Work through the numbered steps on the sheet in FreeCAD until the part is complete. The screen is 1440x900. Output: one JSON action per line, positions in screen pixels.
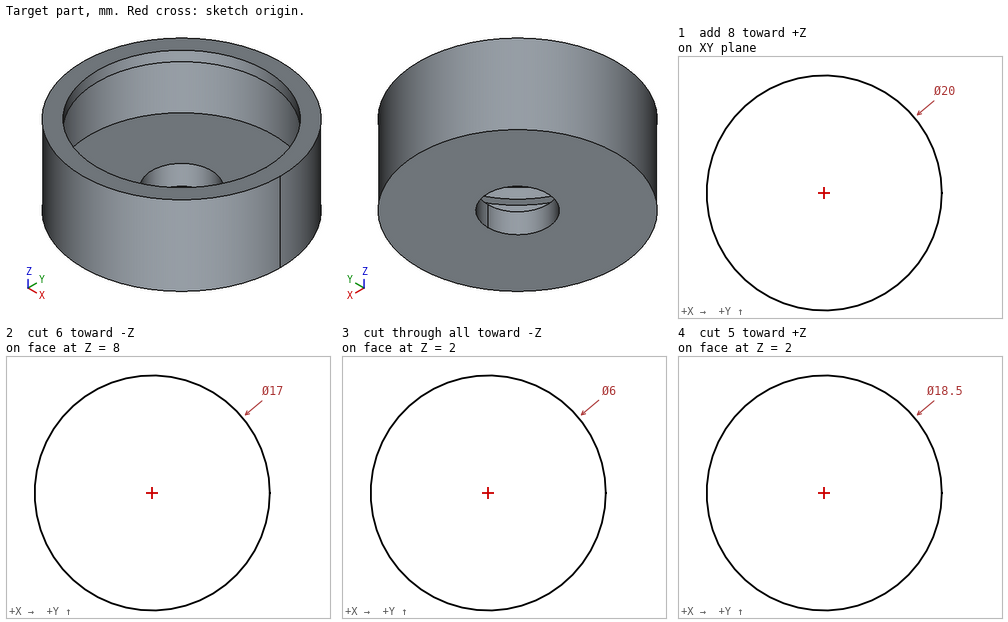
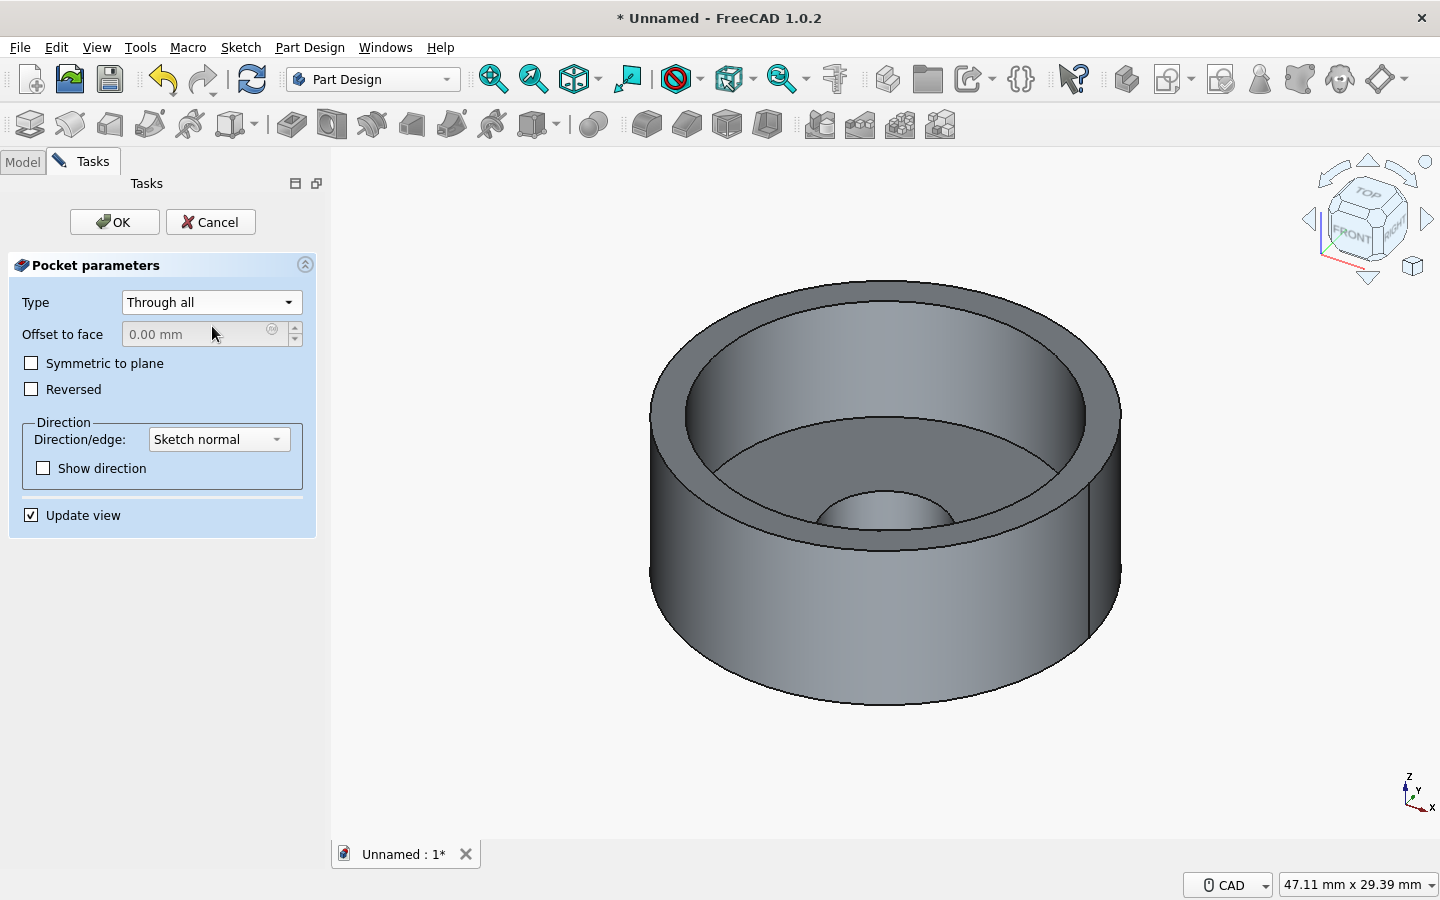
{"action": "left_click", "coordinate": [115, 222]}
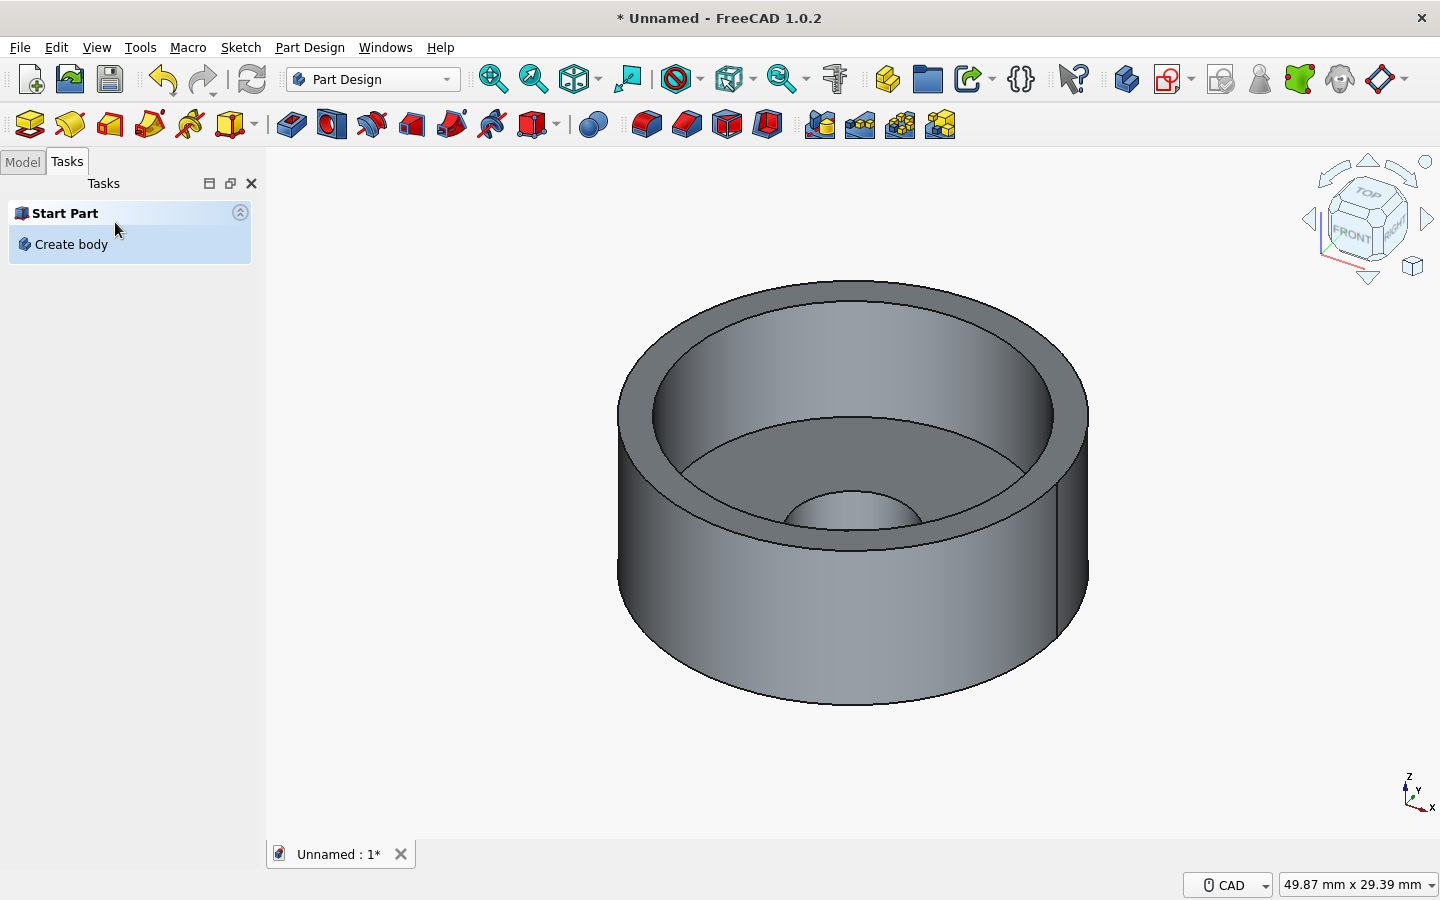
{"action": "left_click", "coordinate": [861, 457]}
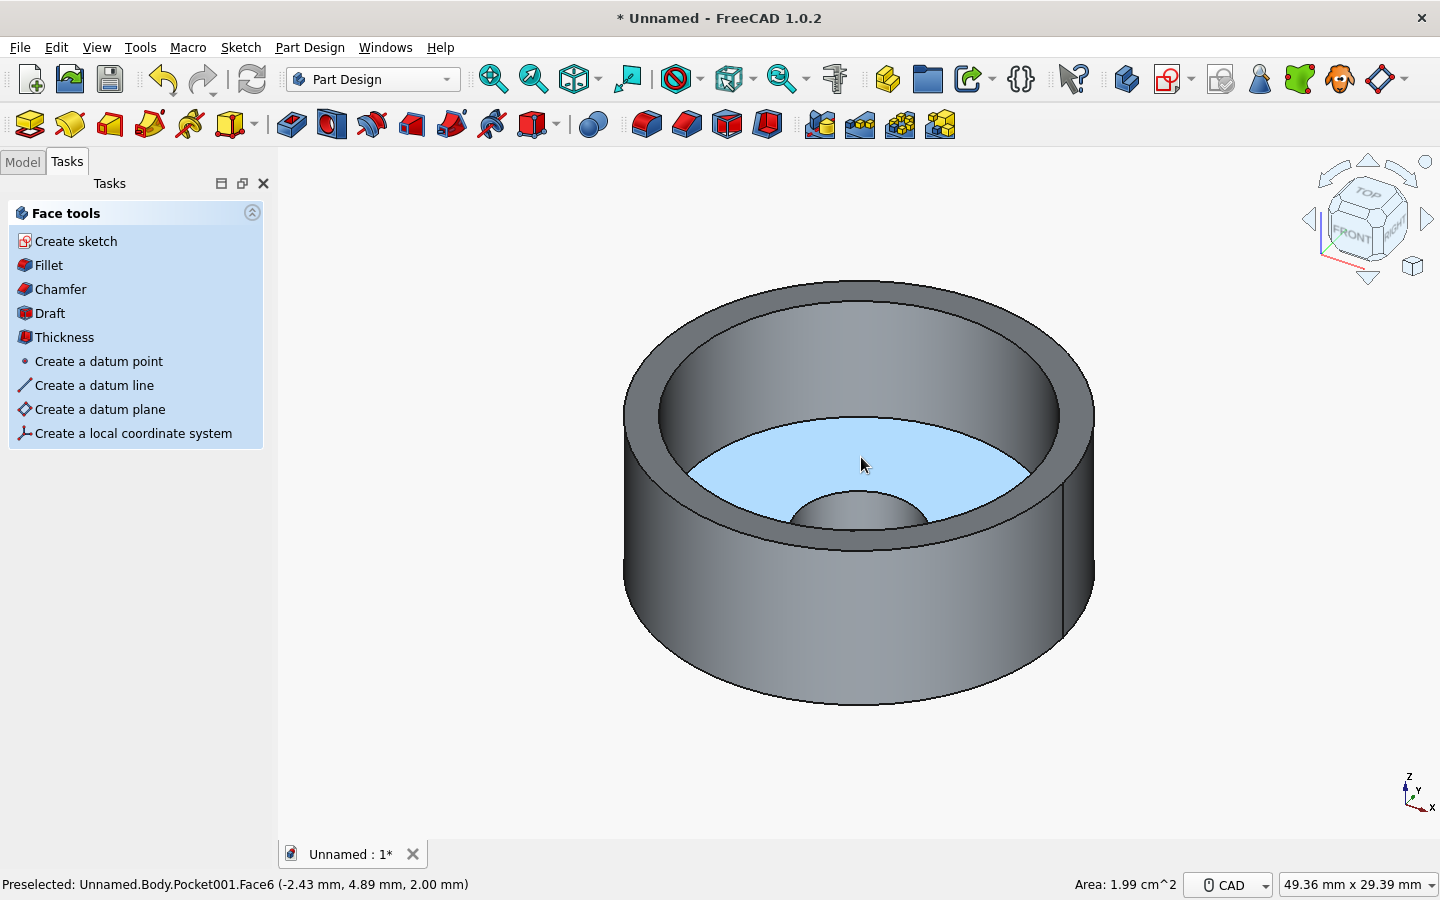
{"action": "left_click", "coordinate": [1168, 80]}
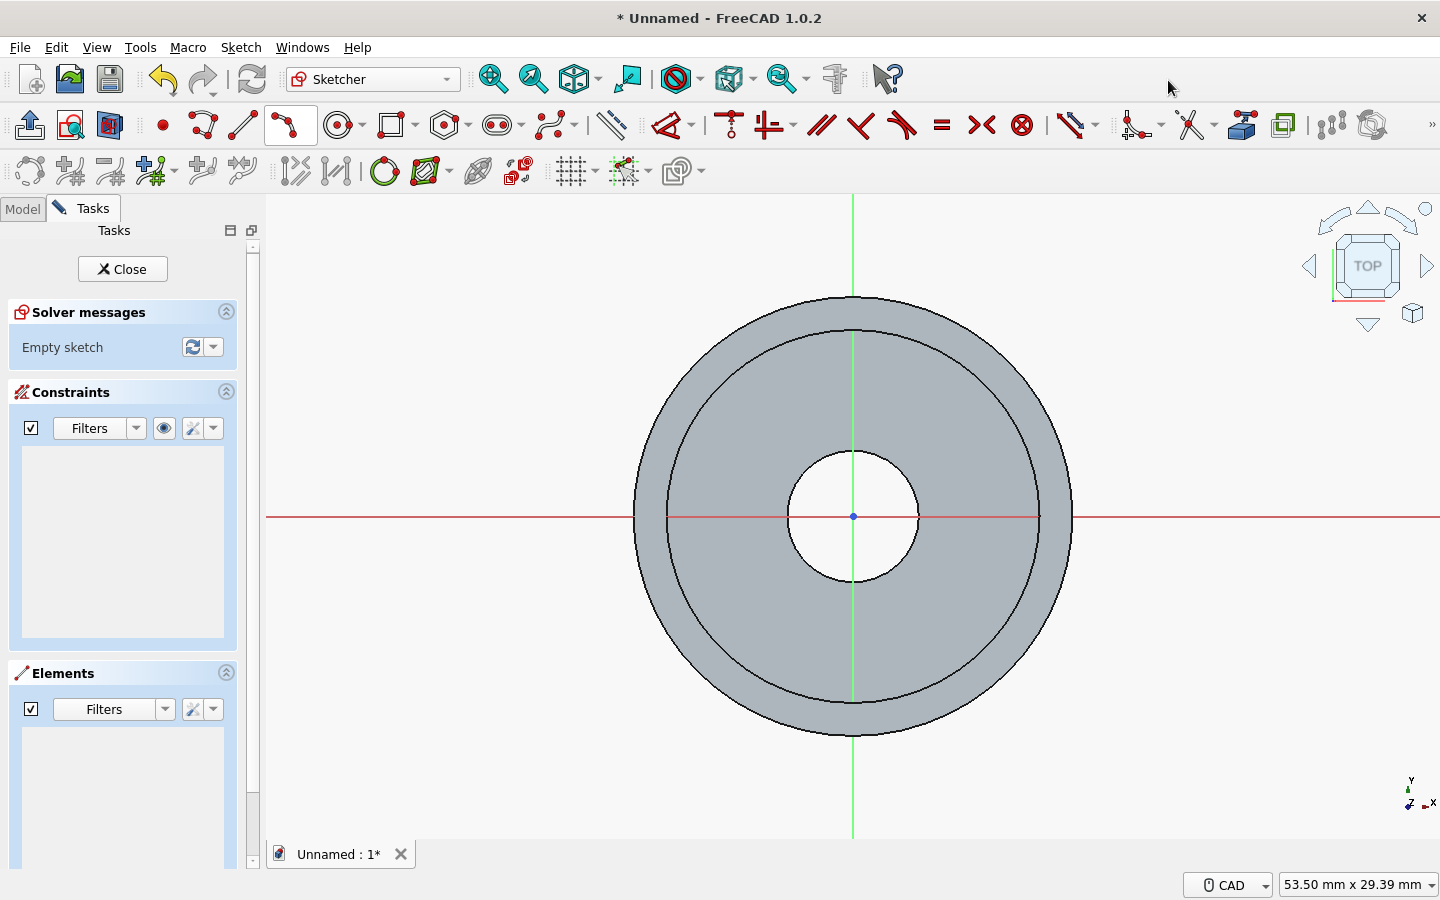
{"action": "key", "text": "q s"}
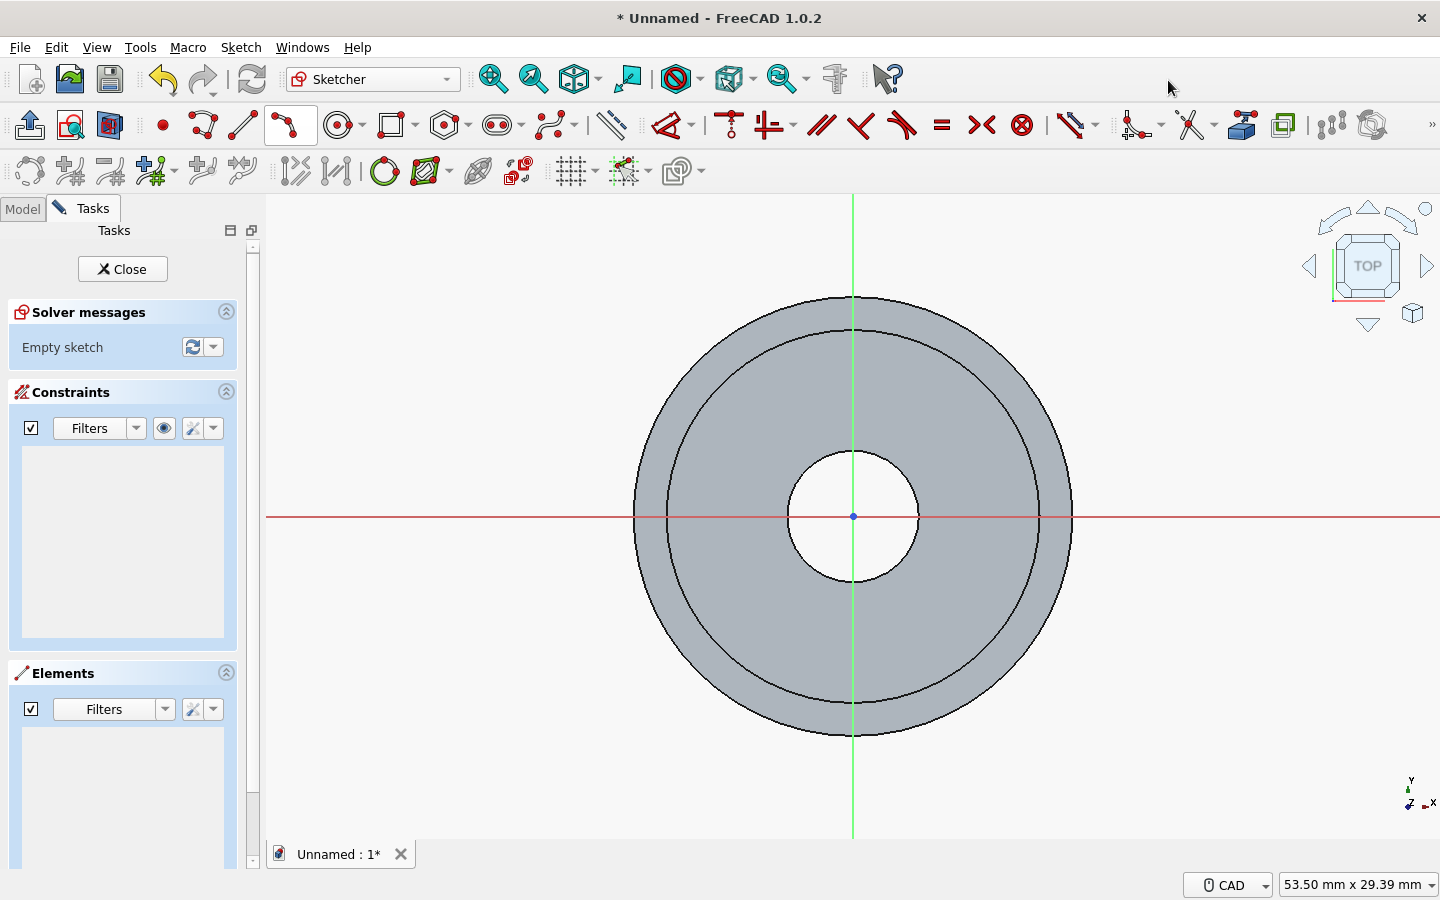
{"action": "left_click", "coordinate": [338, 126]}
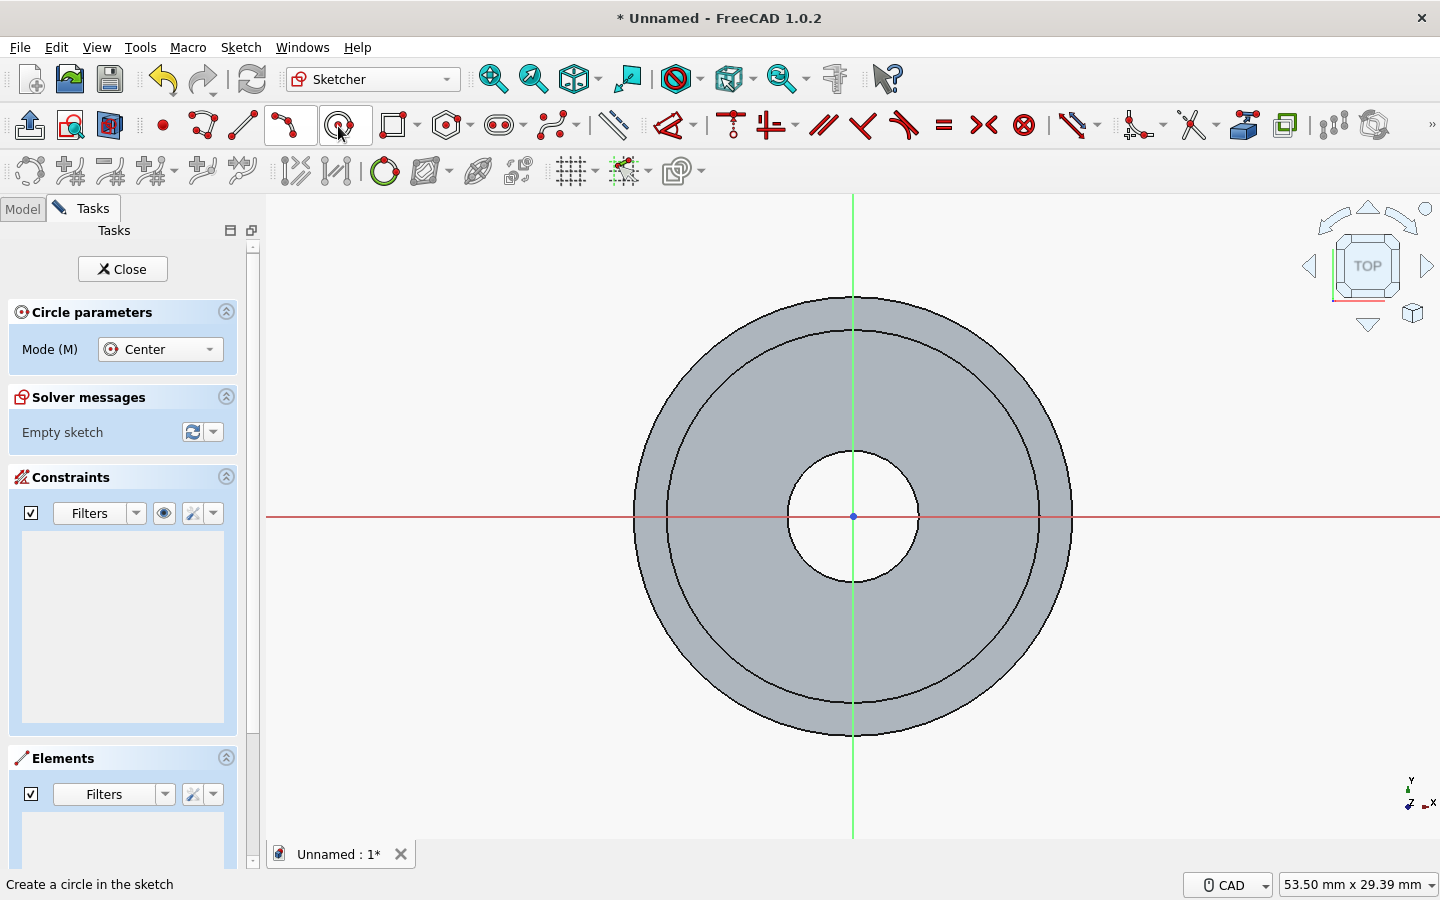
{"action": "left_click", "coordinate": [853, 516]}
{"action": "mouse_move", "coordinate": [997, 373]}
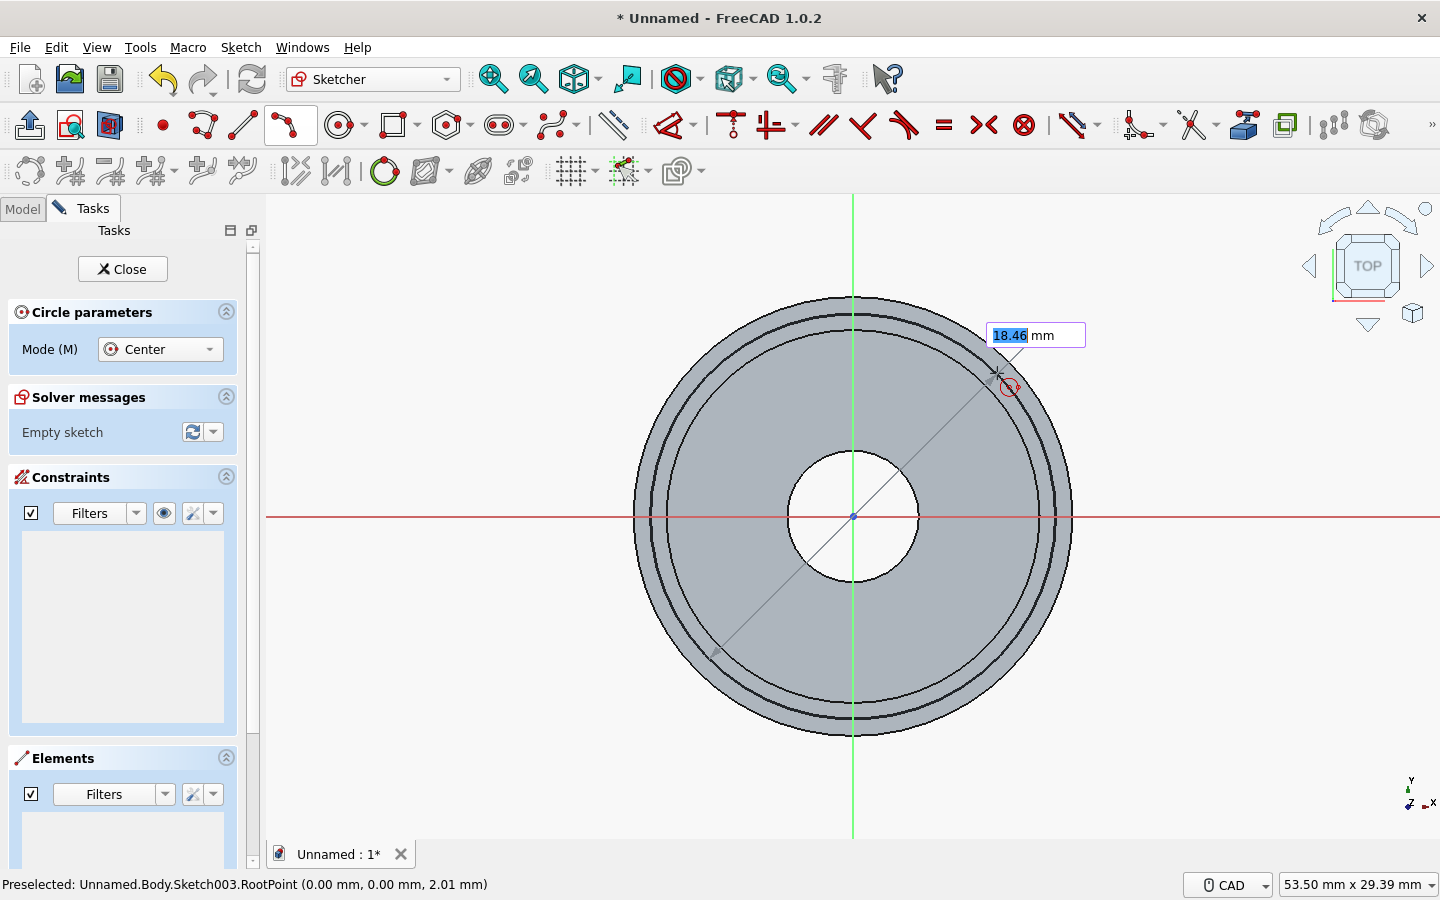
{"action": "type", "text": "18.5"}
{"action": "key", "text": "Return"}
{"action": "key", "text": "Escape"}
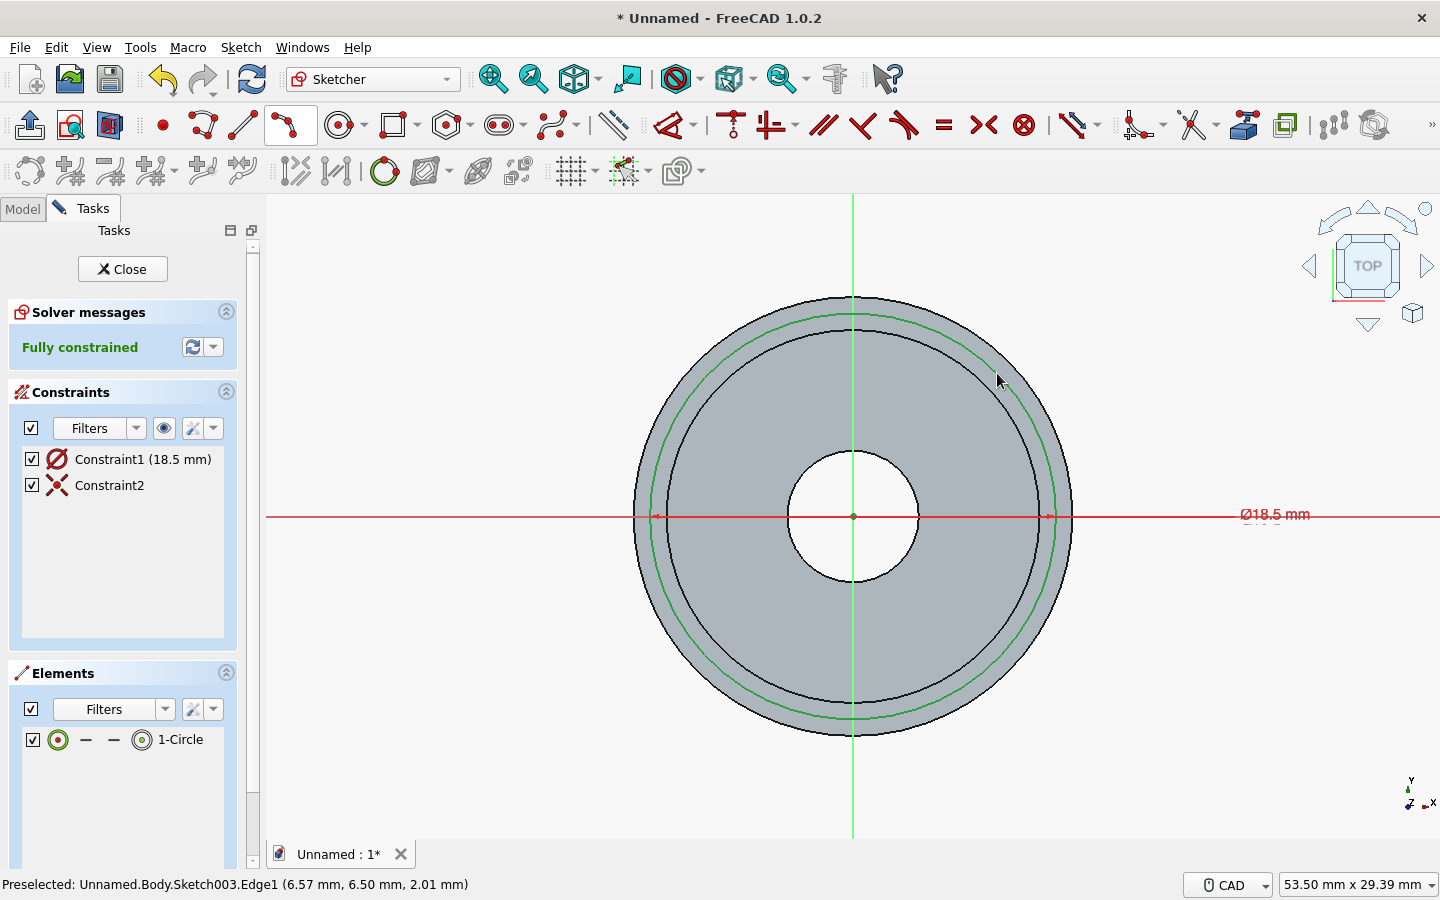
{"action": "left_click", "coordinate": [123, 269]}